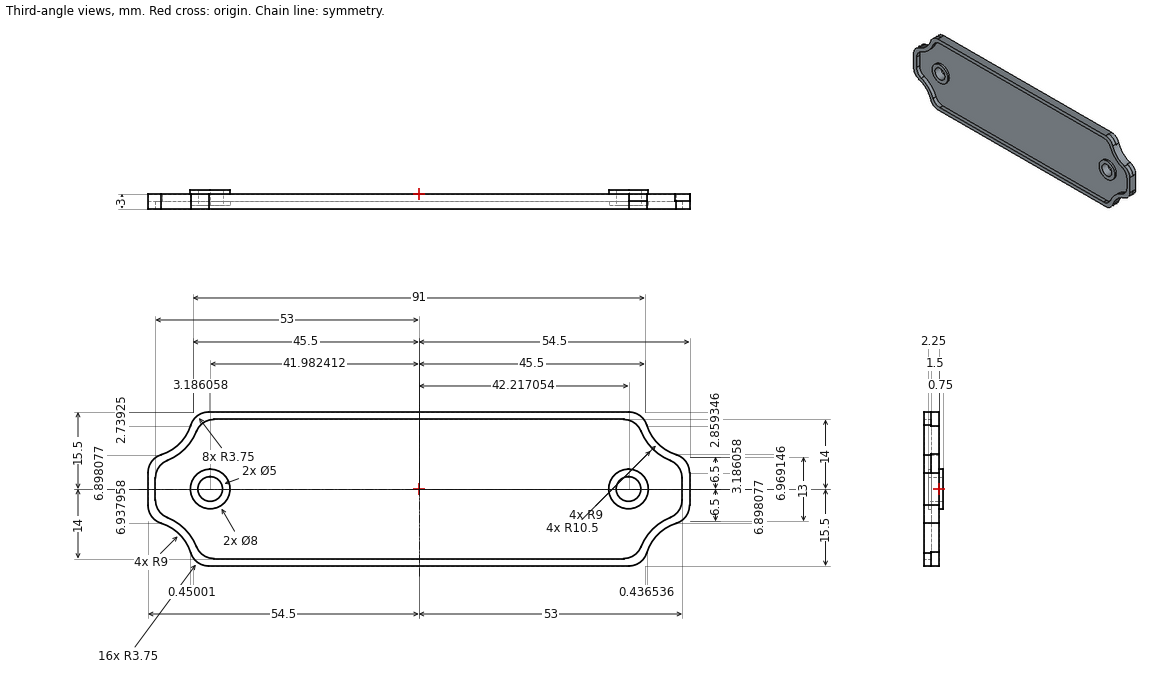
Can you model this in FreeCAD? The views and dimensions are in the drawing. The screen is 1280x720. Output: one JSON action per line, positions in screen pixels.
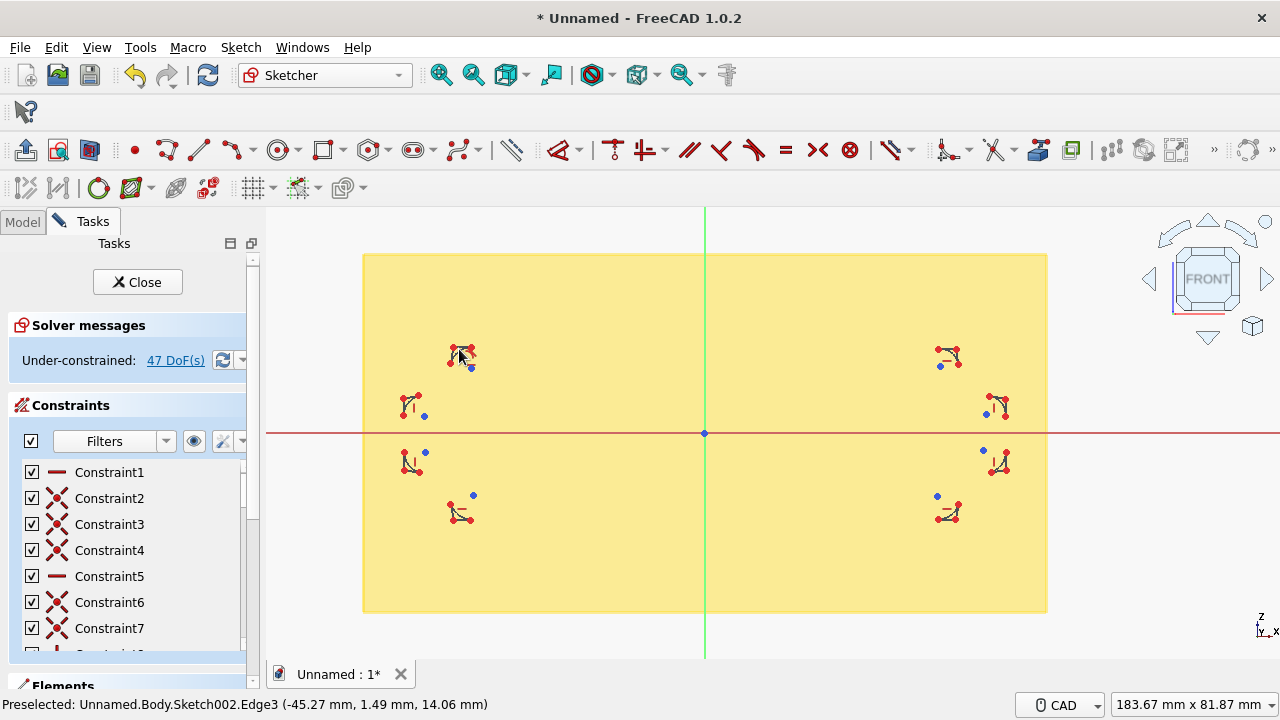
{"action": "scroll", "coordinate": [951, 349], "scroll_direction": "up", "scroll_amount": 9}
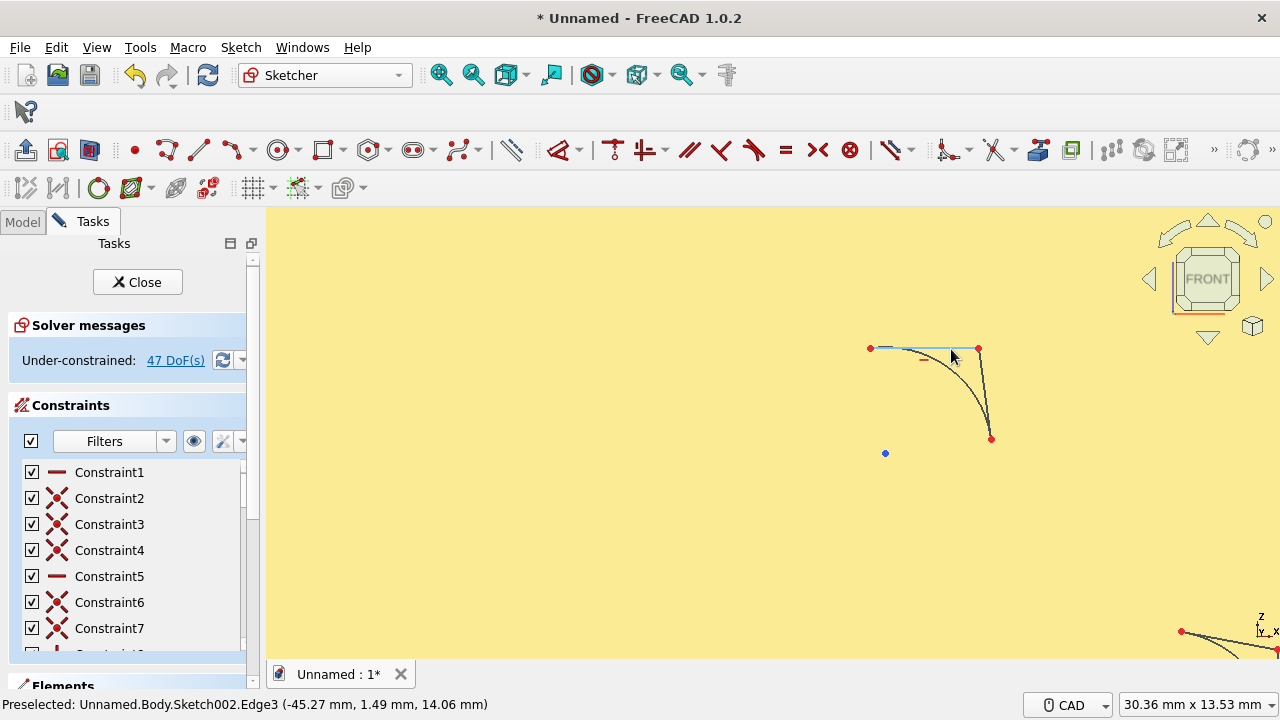
{"action": "left_click", "coordinate": [946, 348]}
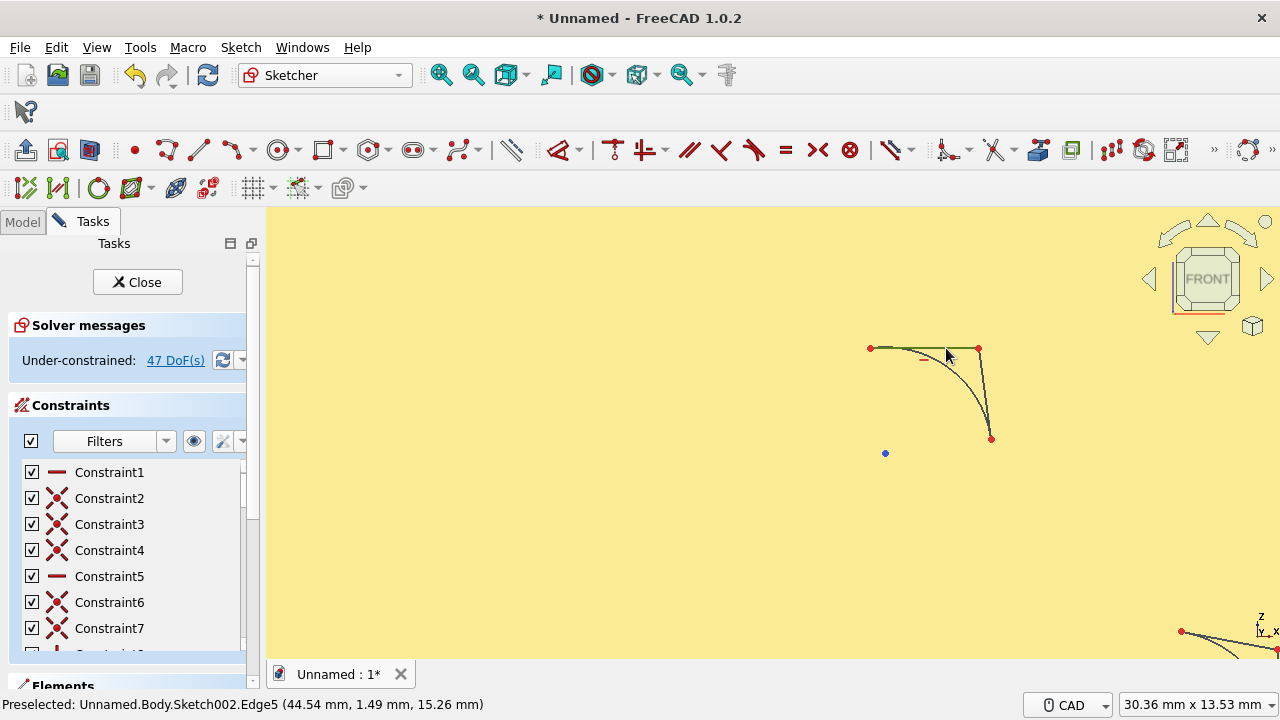
{"action": "left_click", "coordinate": [973, 393]}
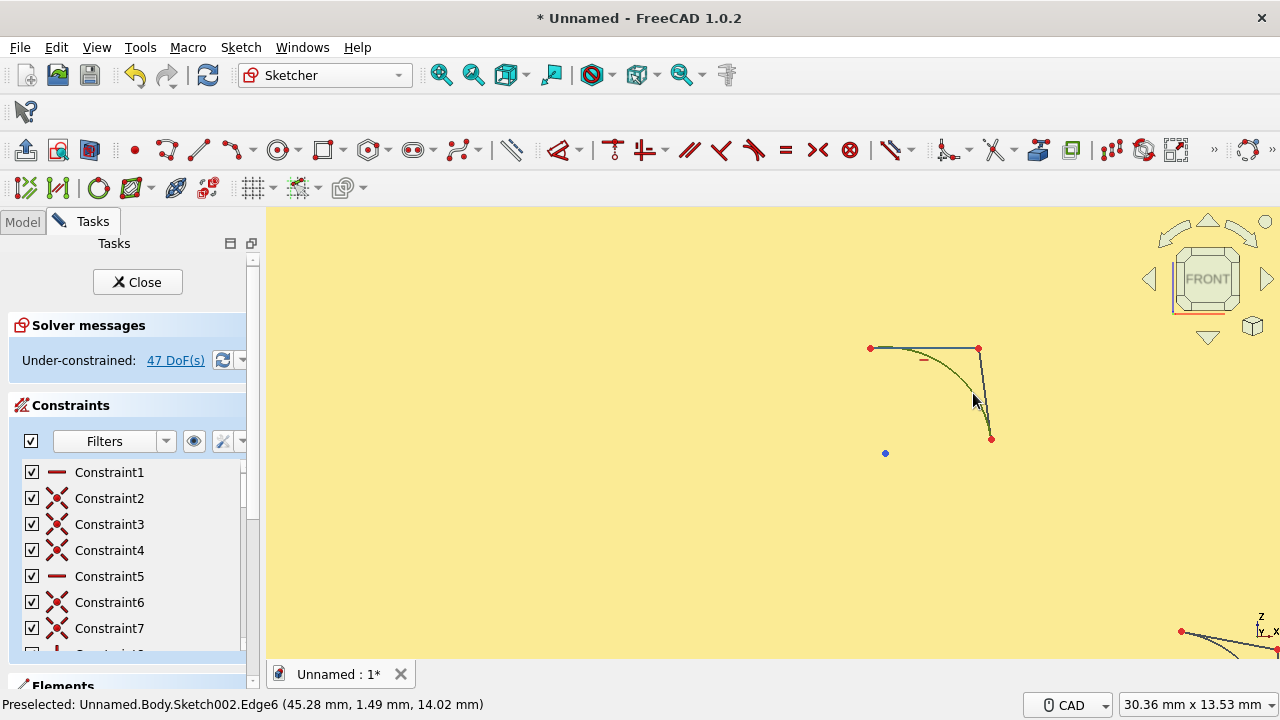
{"action": "left_click", "coordinate": [754, 150]}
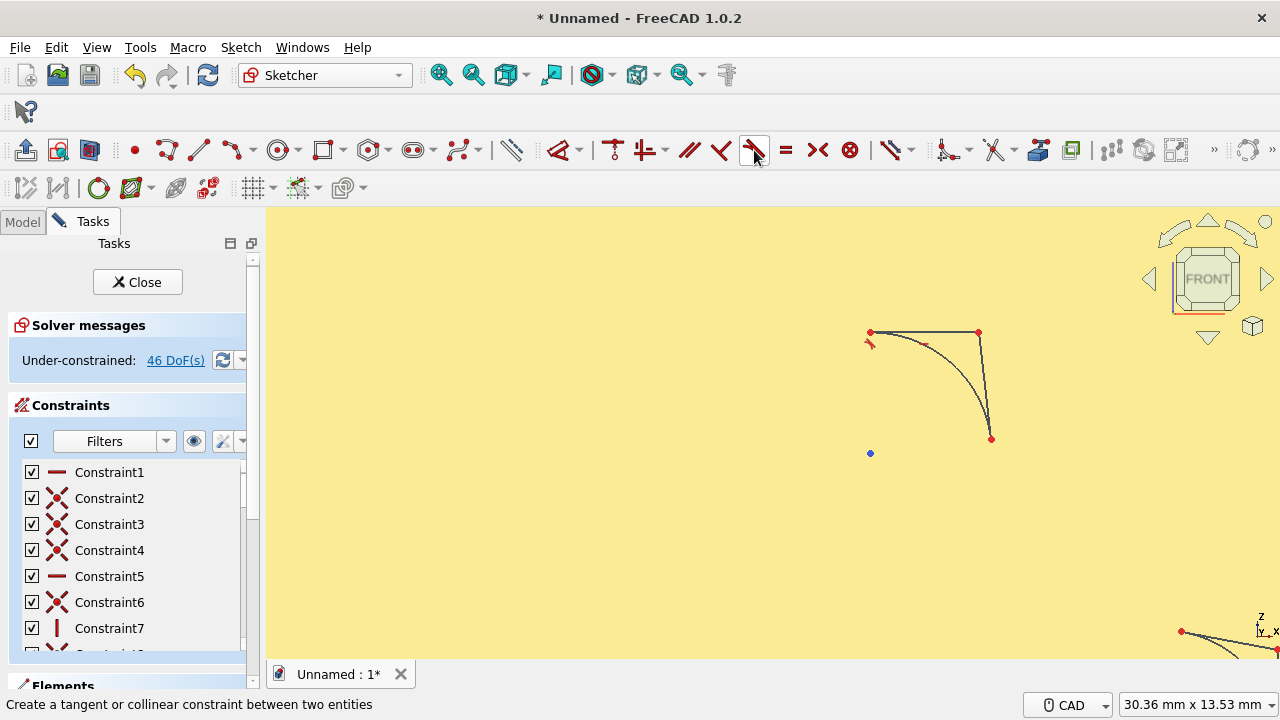
{"action": "scroll", "coordinate": [951, 349], "scroll_direction": "down", "scroll_amount": 9}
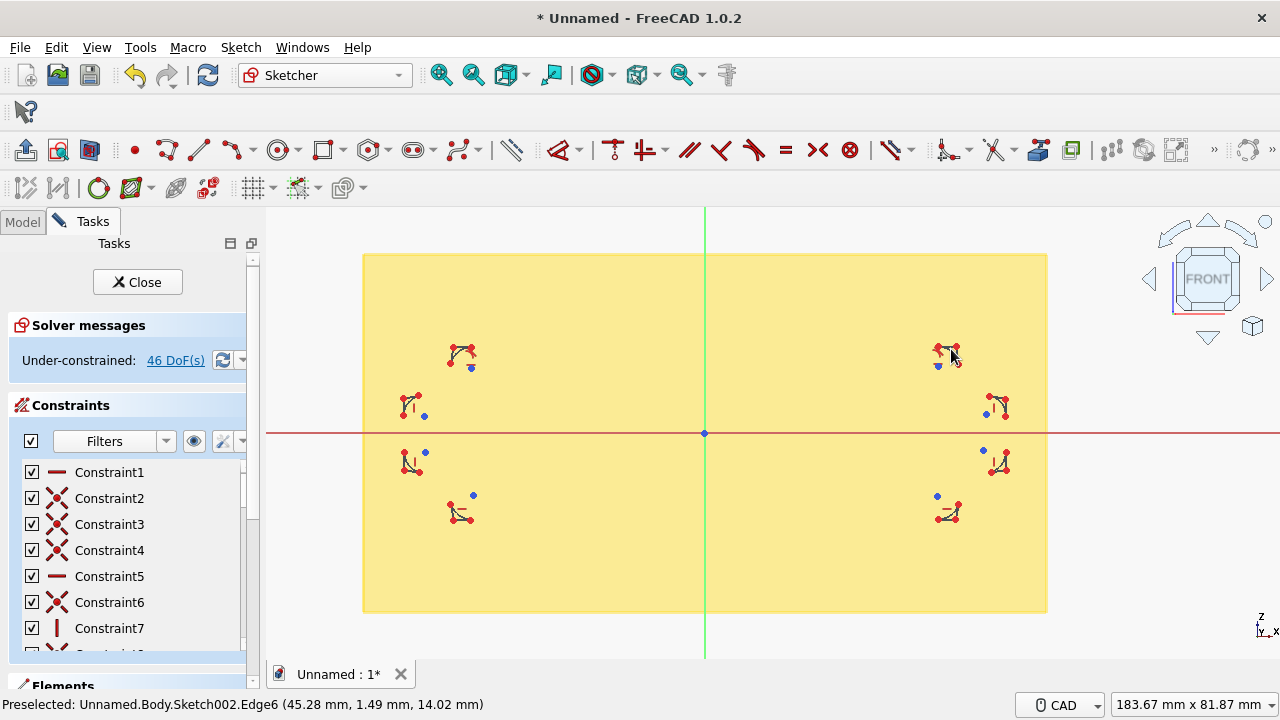
{"action": "scroll", "coordinate": [1006, 404], "scroll_direction": "up", "scroll_amount": 9}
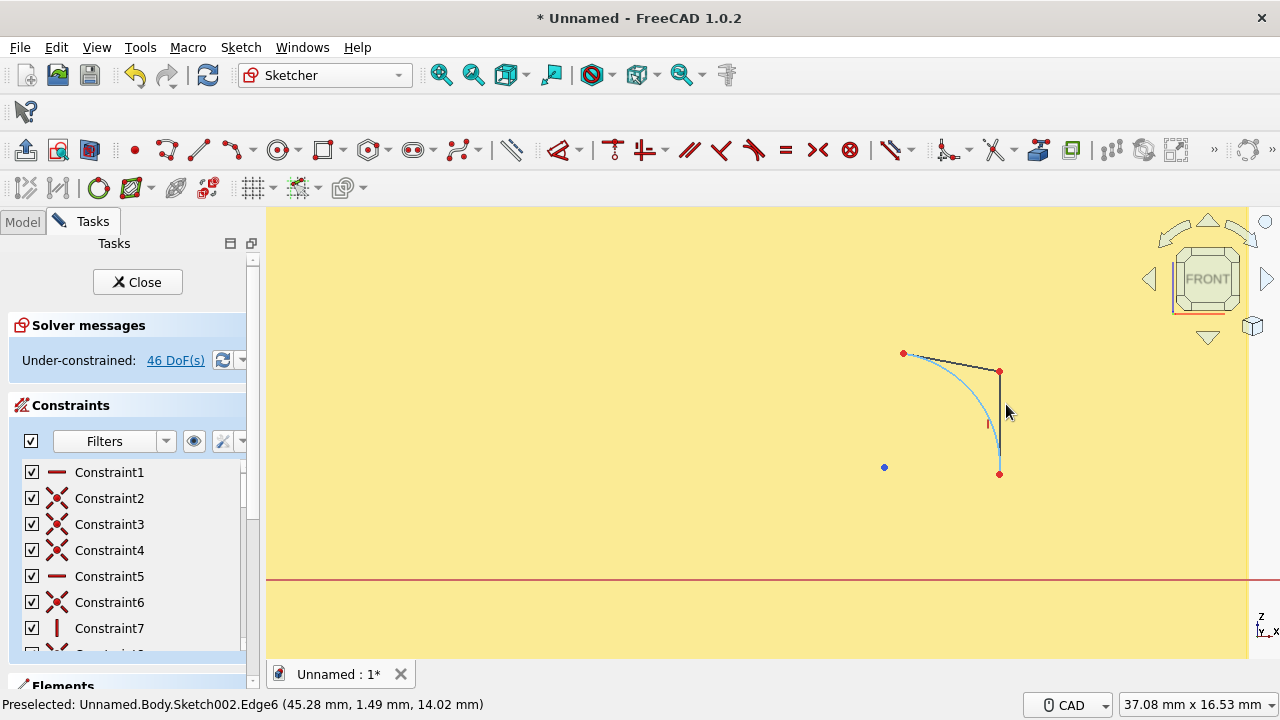
{"action": "left_click", "coordinate": [1000, 402]}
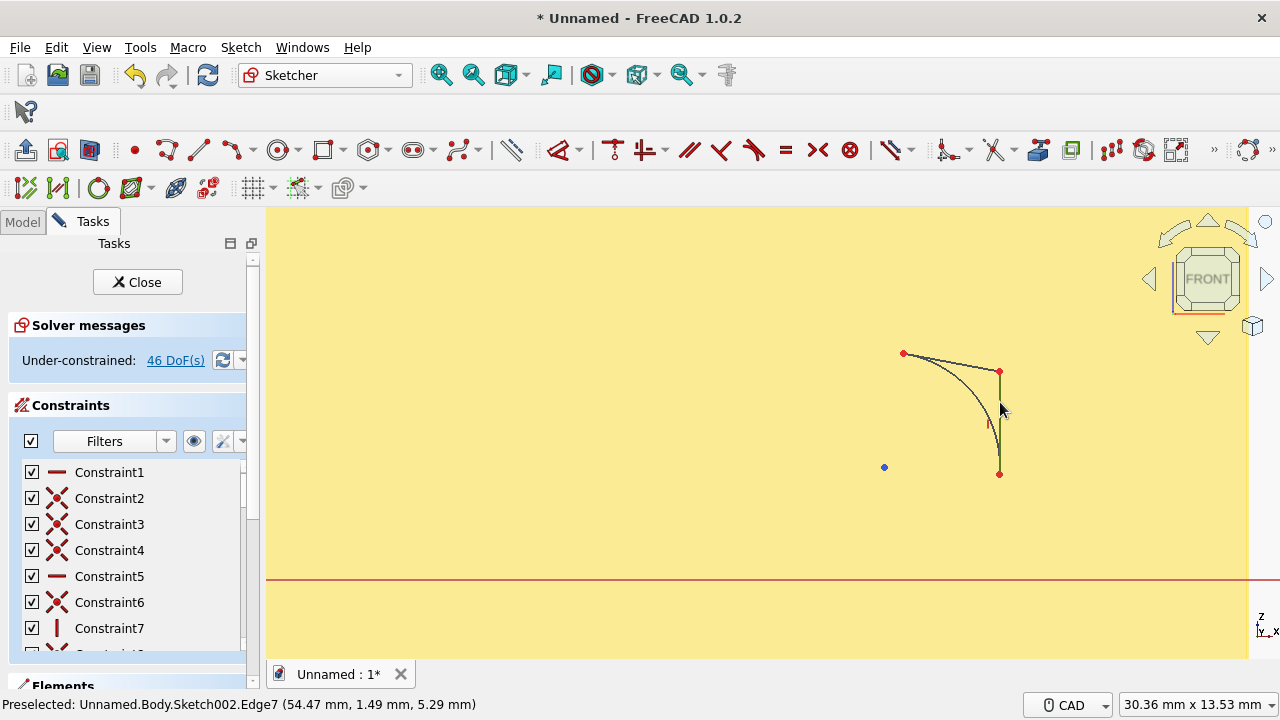
{"action": "scroll", "coordinate": [950, 372], "scroll_direction": "up", "scroll_amount": 2}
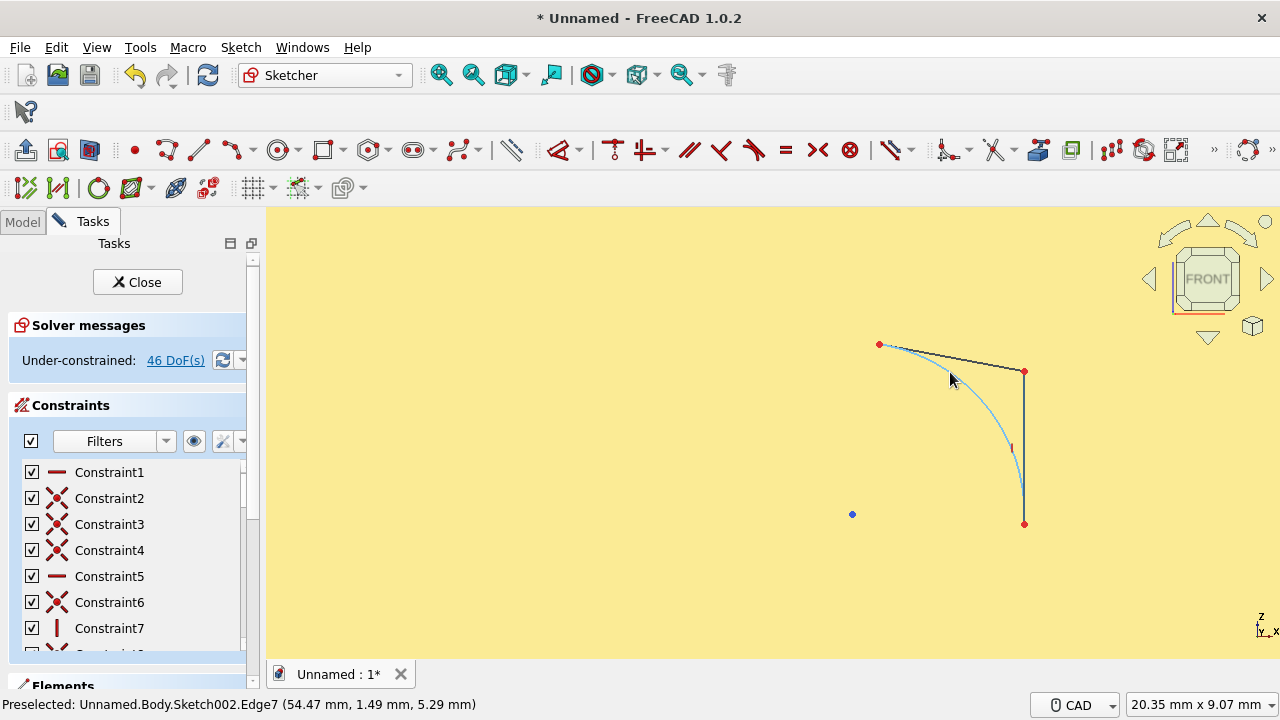
{"action": "left_click", "coordinate": [950, 372]}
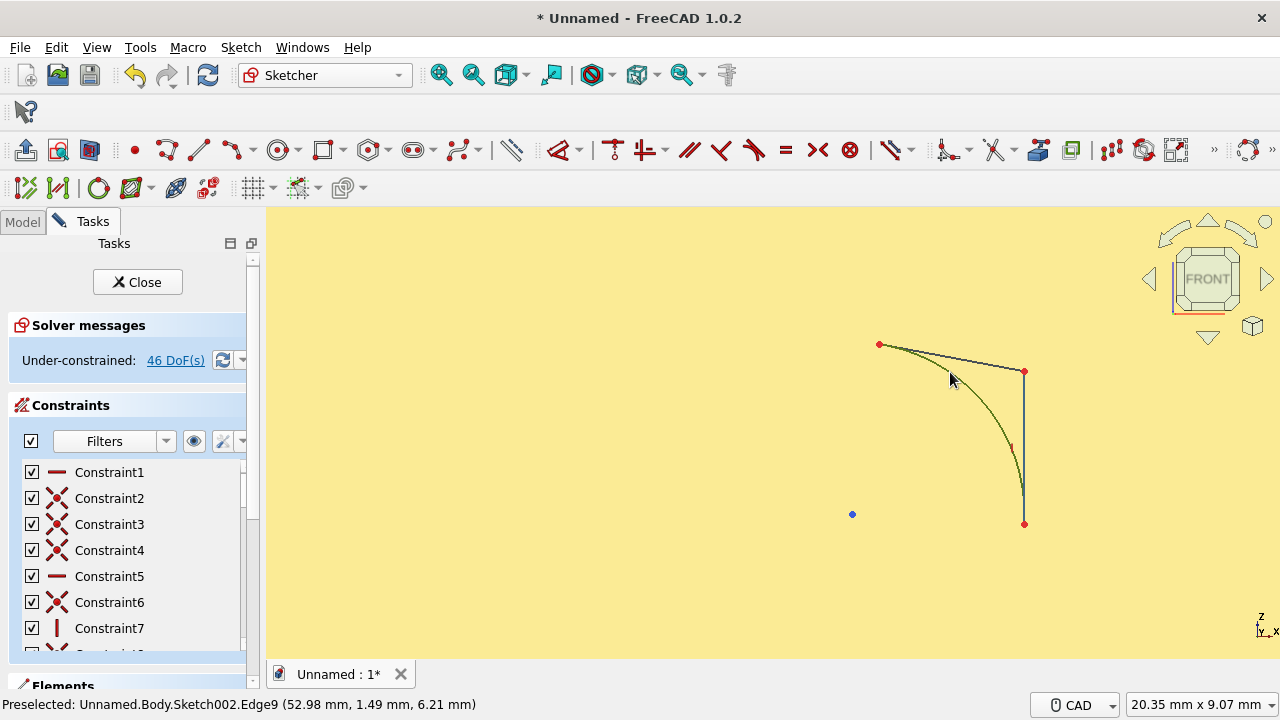
{"action": "left_click", "coordinate": [754, 150]}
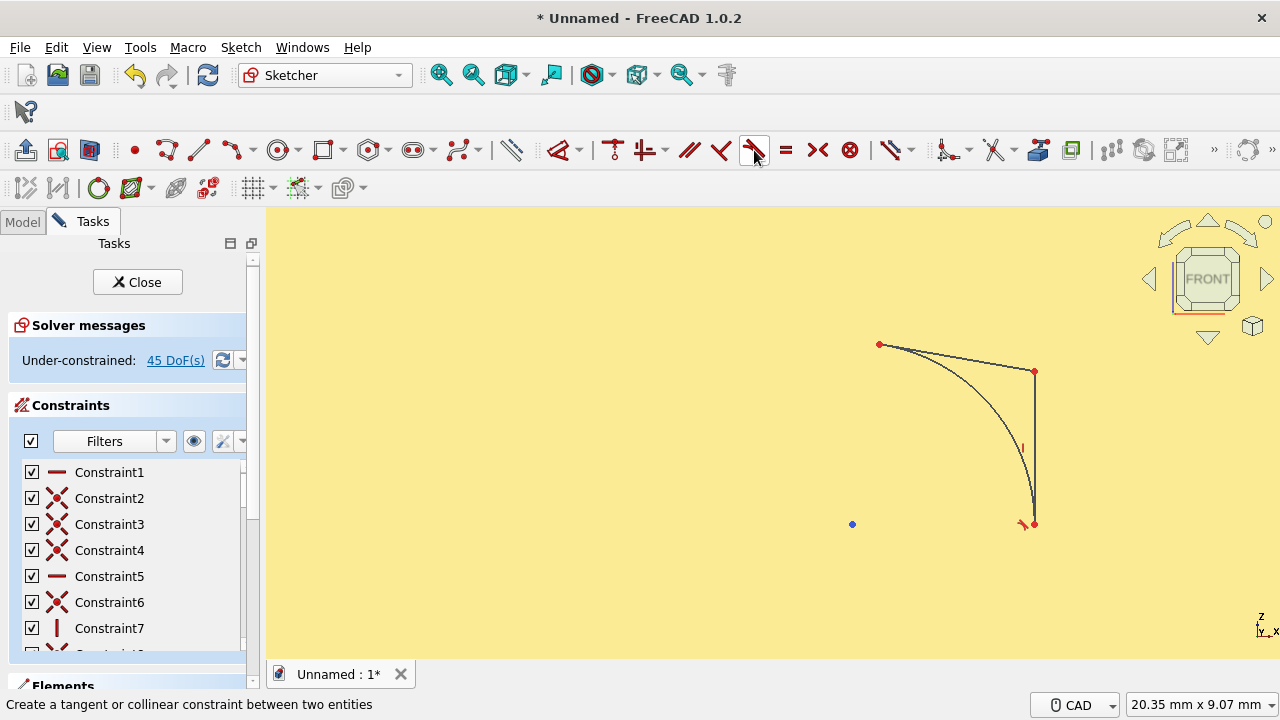
{"action": "scroll", "coordinate": [1003, 402], "scroll_direction": "down", "scroll_amount": 11}